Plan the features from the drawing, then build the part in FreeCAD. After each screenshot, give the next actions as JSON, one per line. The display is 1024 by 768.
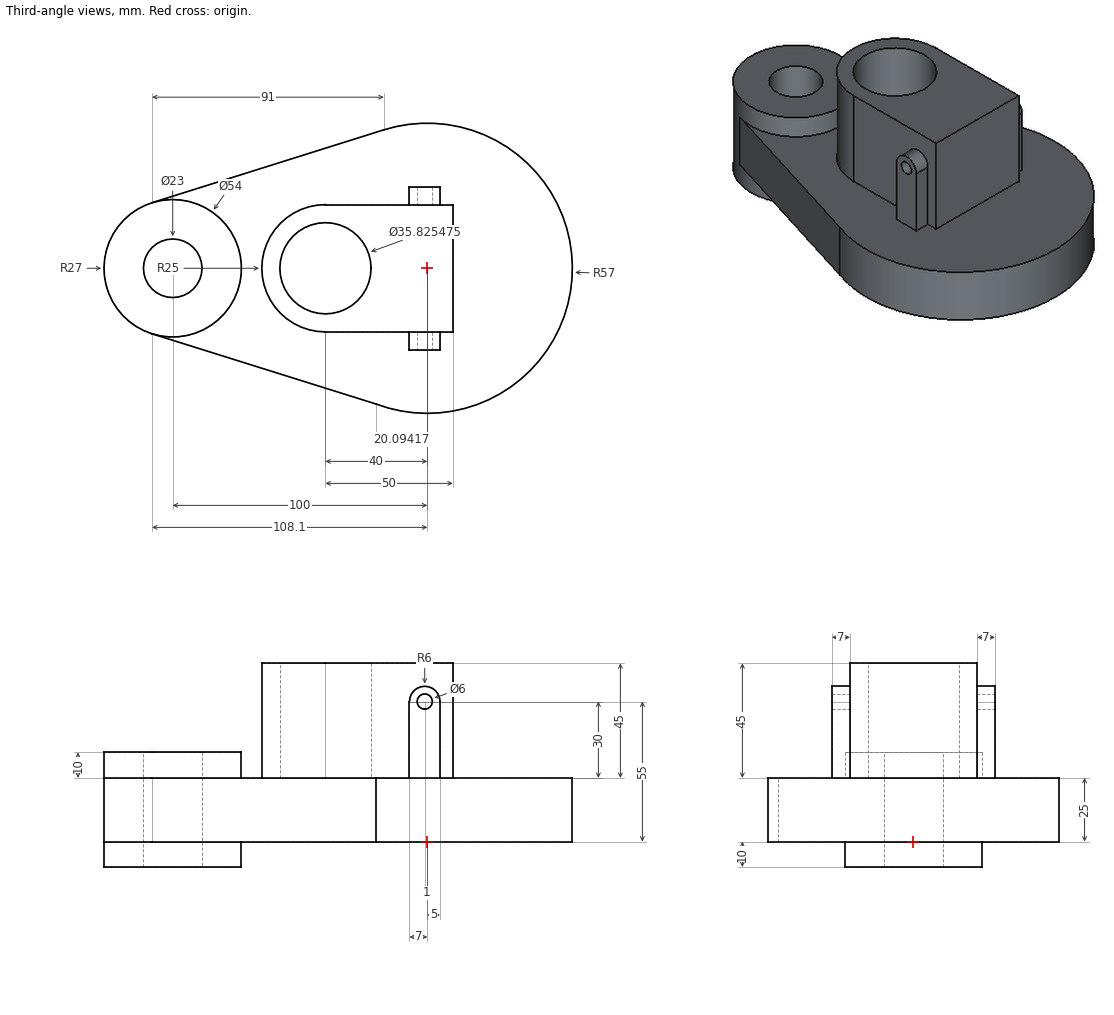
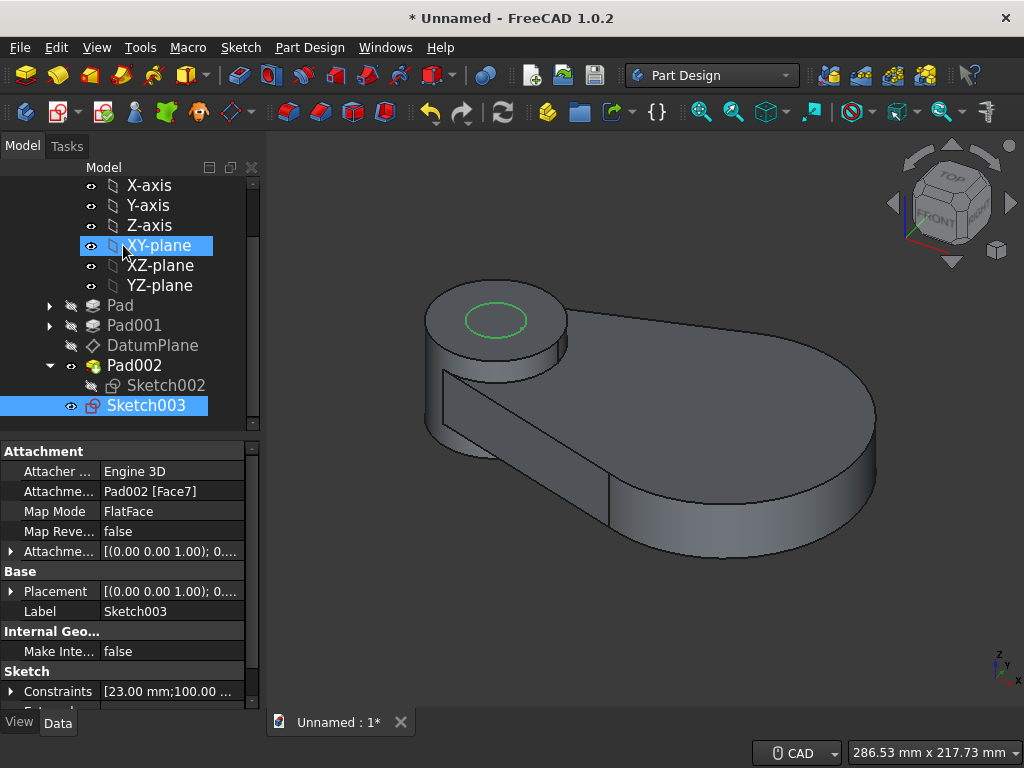
{"action": "left_click", "coordinate": [240, 76]}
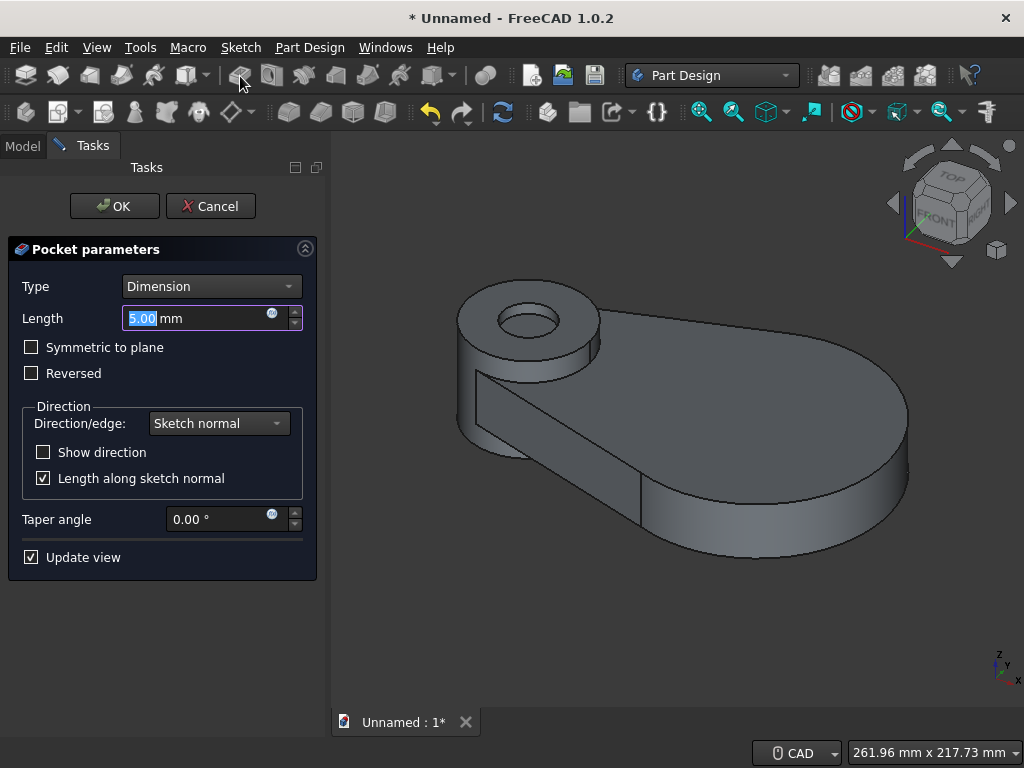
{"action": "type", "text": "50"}
{"action": "key", "text": "Tab"}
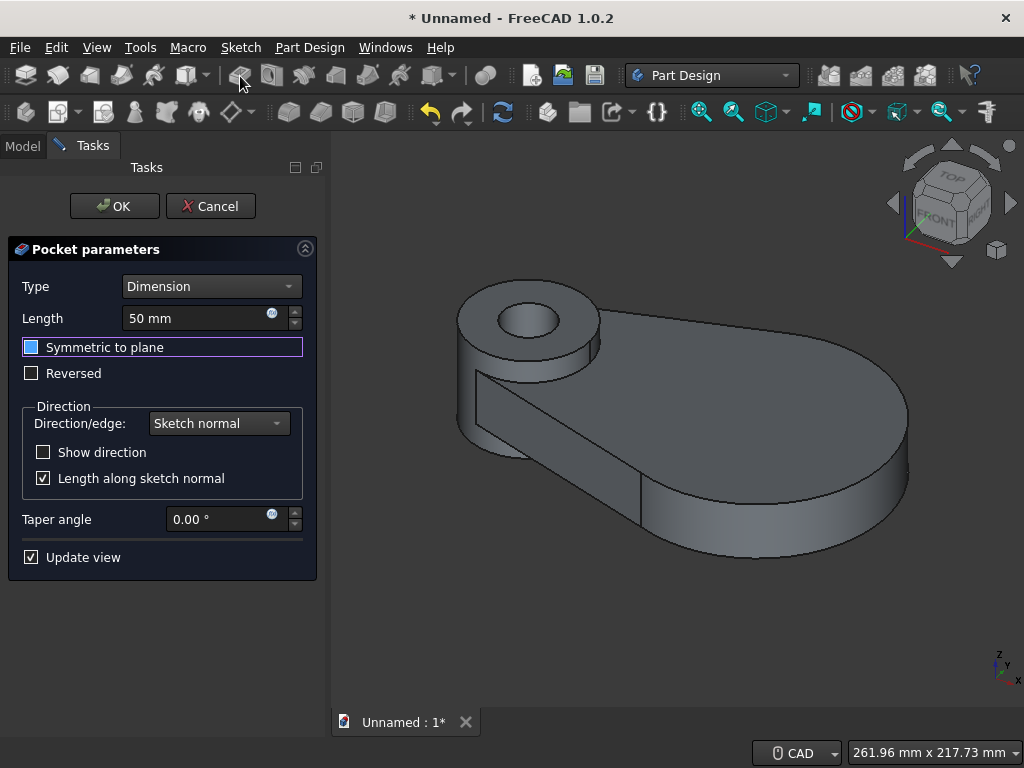
{"action": "left_click", "coordinate": [115, 206]}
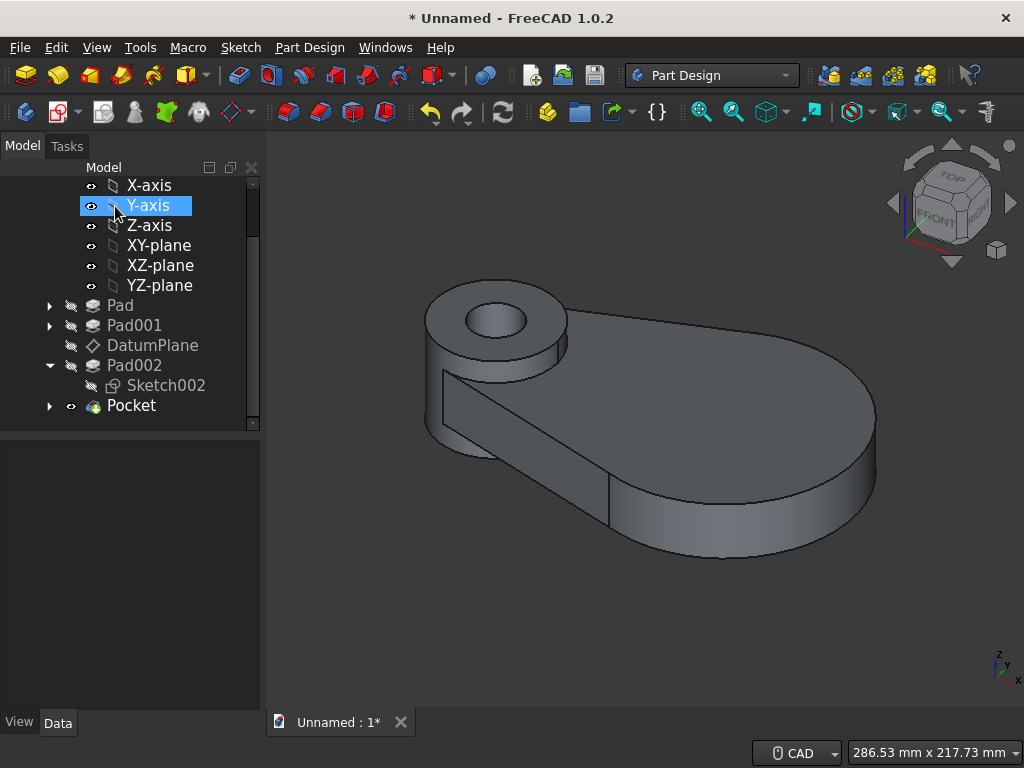
{"action": "left_click", "coordinate": [721, 415]}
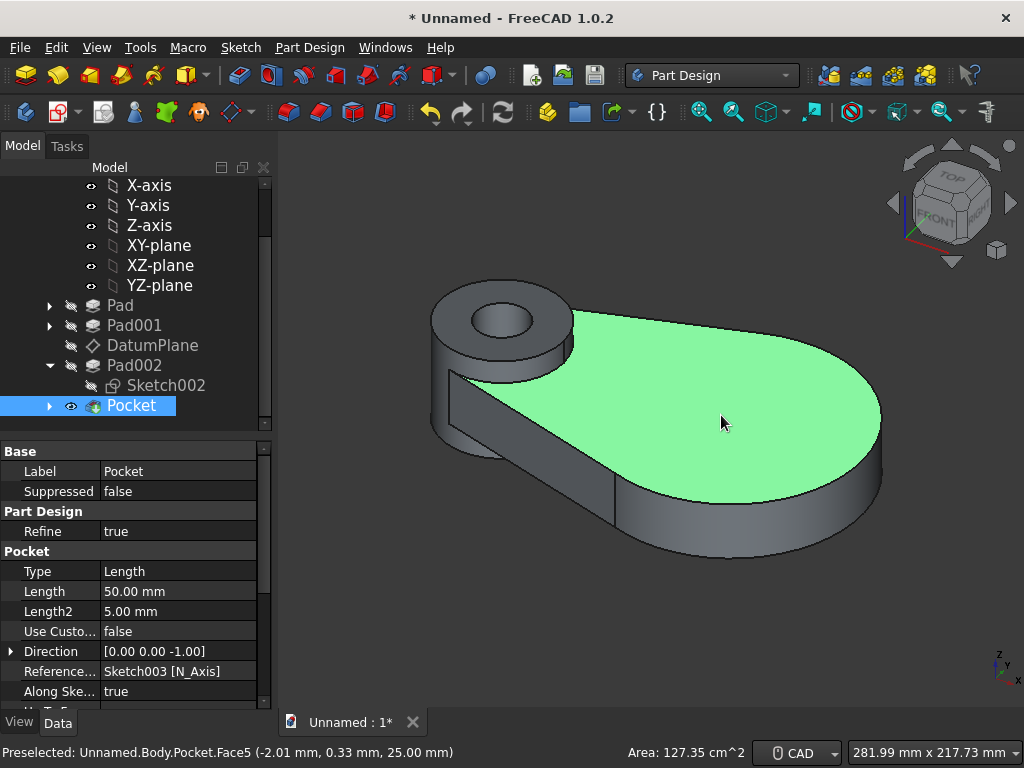
{"action": "left_click", "coordinate": [58, 112]}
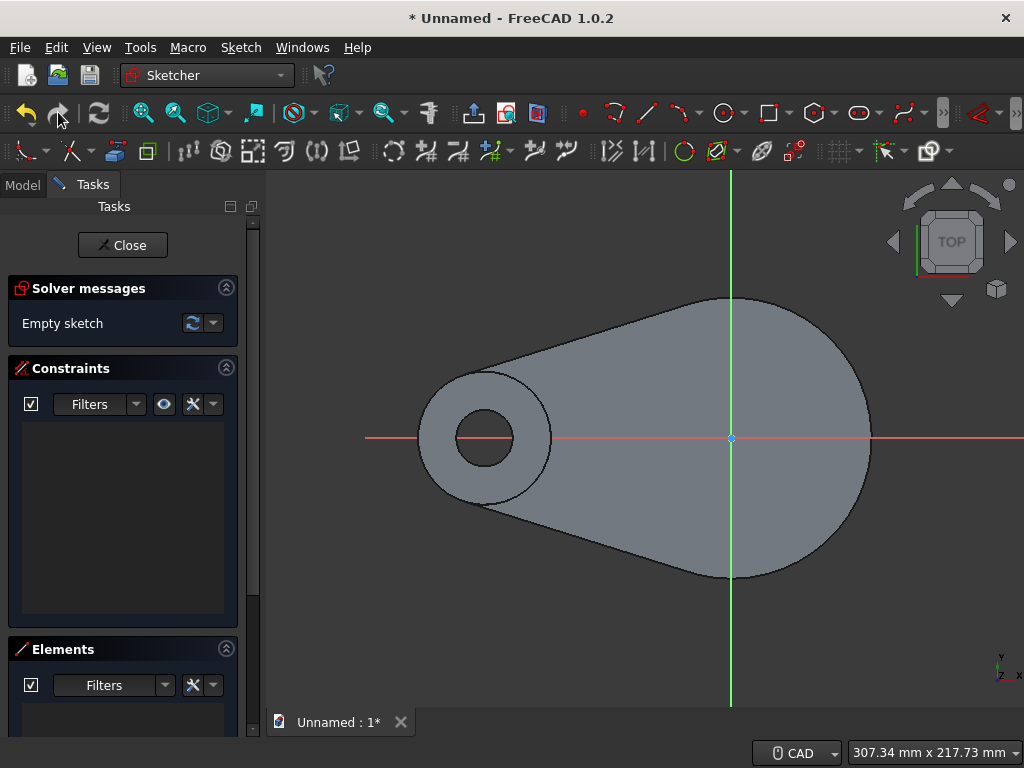
{"action": "scroll", "coordinate": [734, 438], "scroll_direction": "up", "scroll_amount": 4}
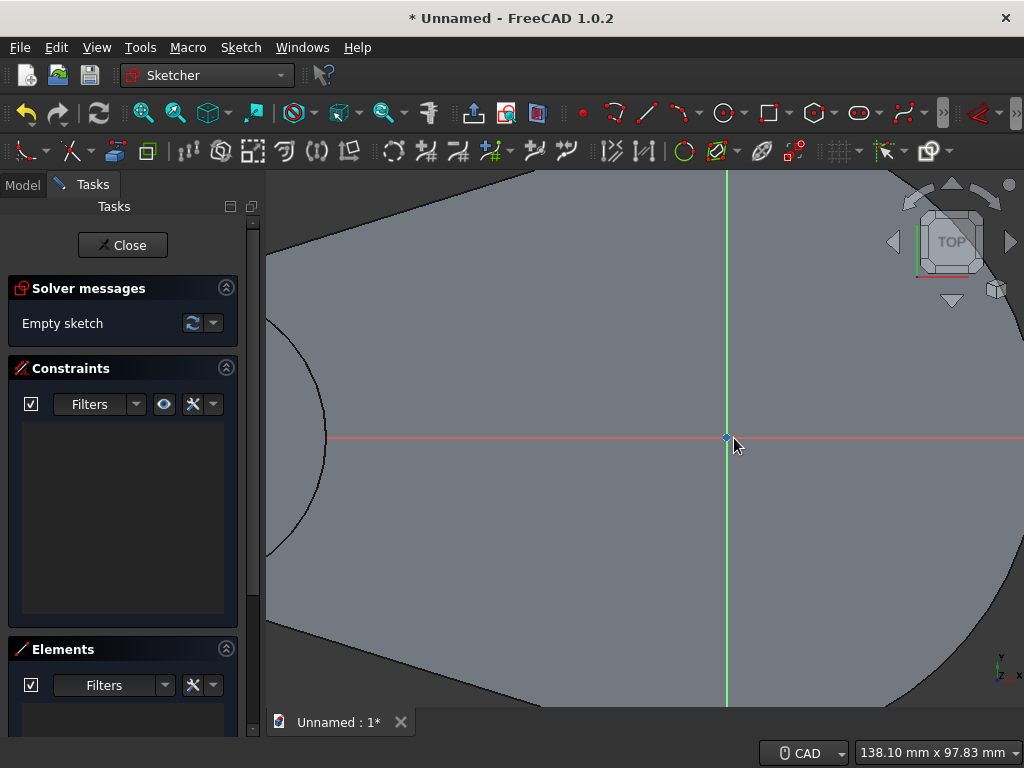
{"action": "key", "text": "g m"}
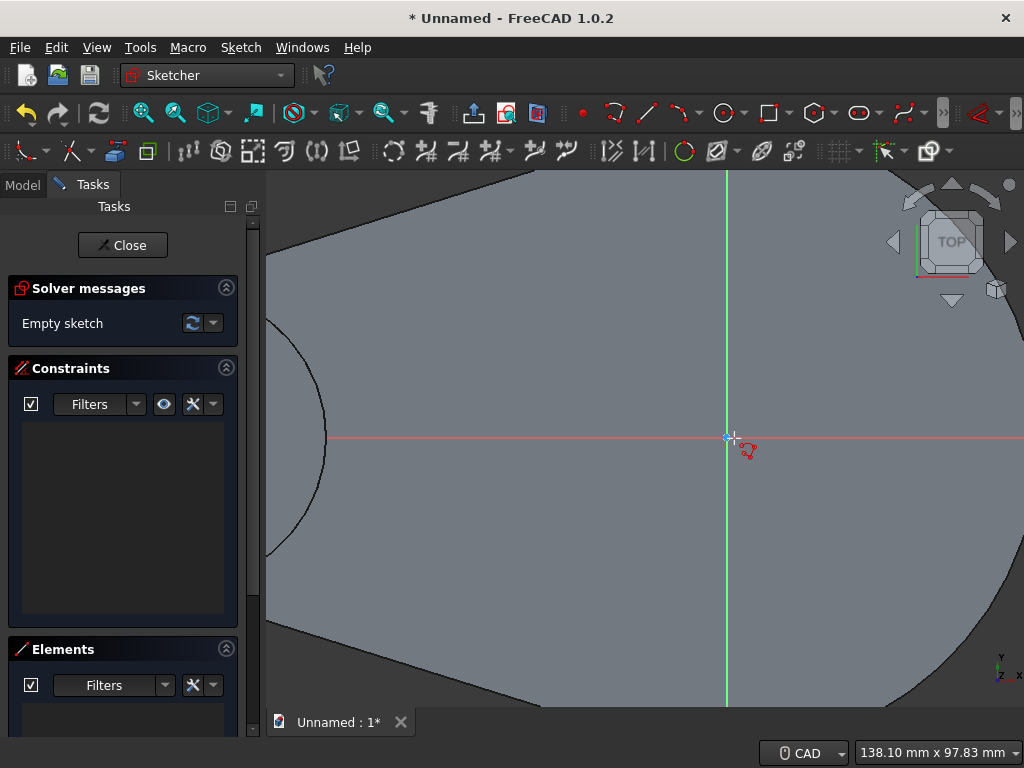
{"action": "left_click", "coordinate": [507, 575]}
{"action": "left_click", "coordinate": [782, 575]}
{"action": "left_click", "coordinate": [782, 301]}
{"action": "left_click", "coordinate": [507, 301]}
{"action": "right_click", "coordinate": [507, 301]}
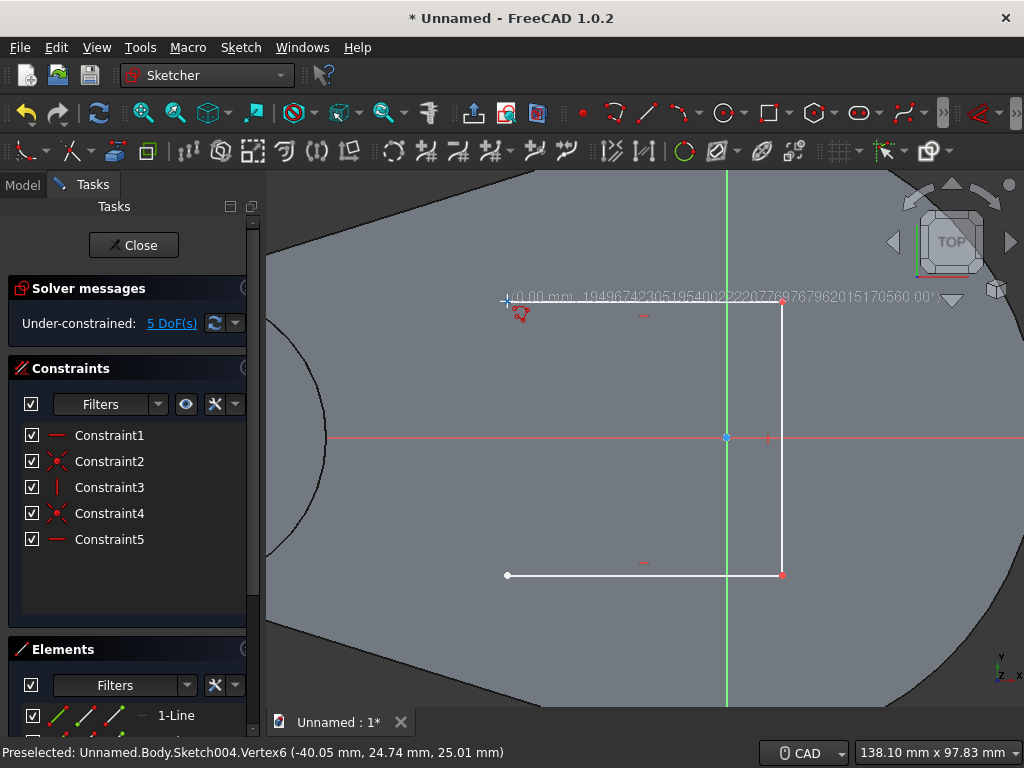
{"action": "left_click", "coordinate": [680, 114]}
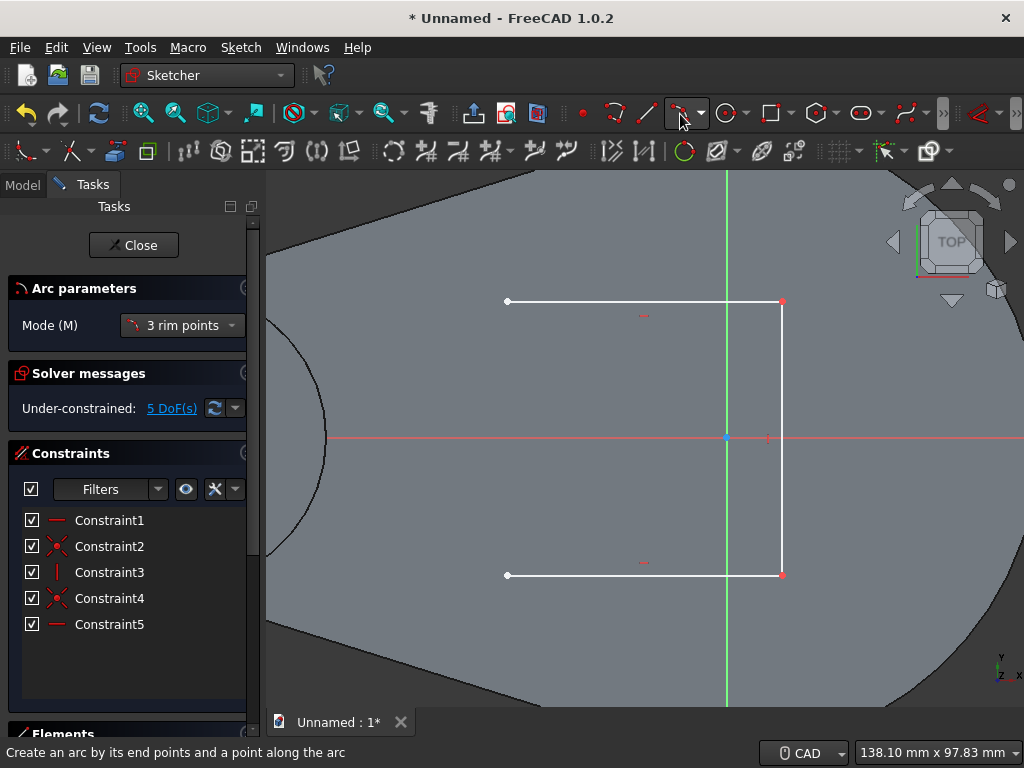
{"action": "left_click", "coordinate": [507, 302]}
{"action": "left_click", "coordinate": [507, 576]}
{"action": "left_click", "coordinate": [377, 395]}
{"action": "key", "text": "Escape"}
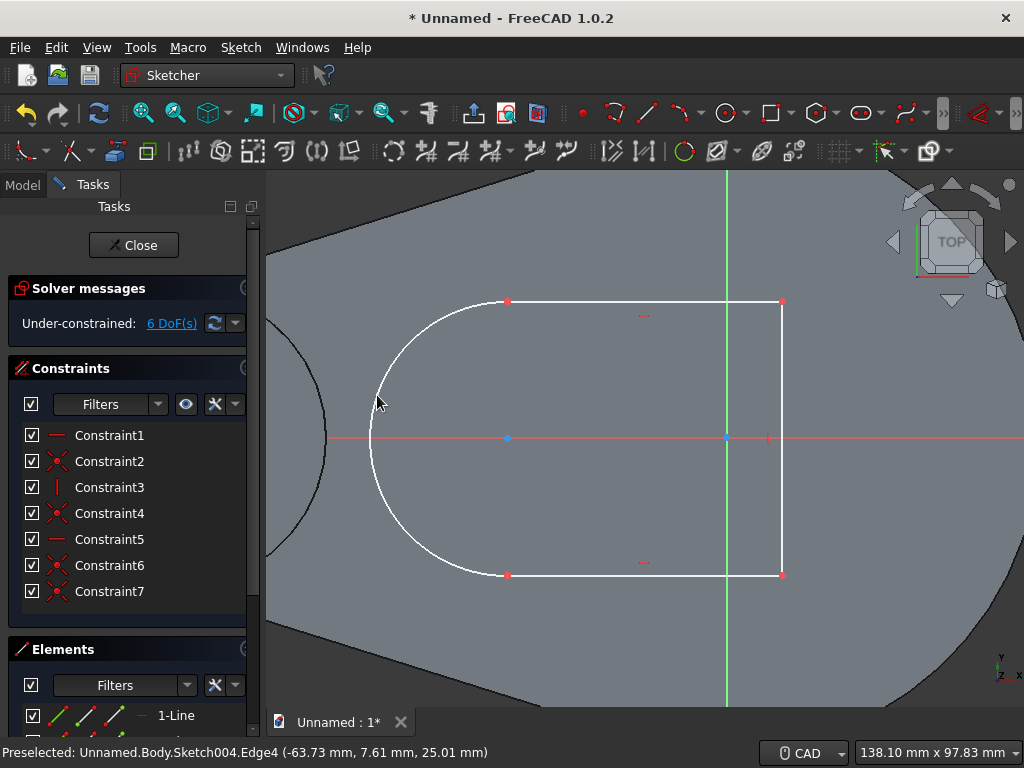
{"action": "left_click", "coordinate": [590, 576]}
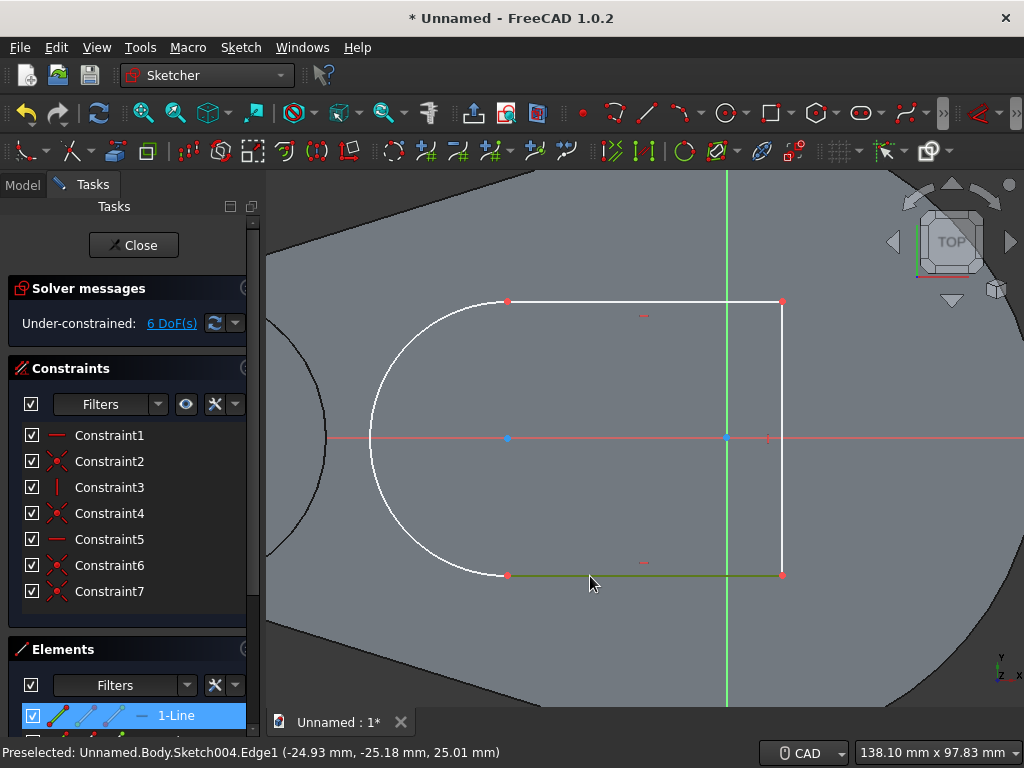
{"action": "left_click", "coordinate": [396, 358]}